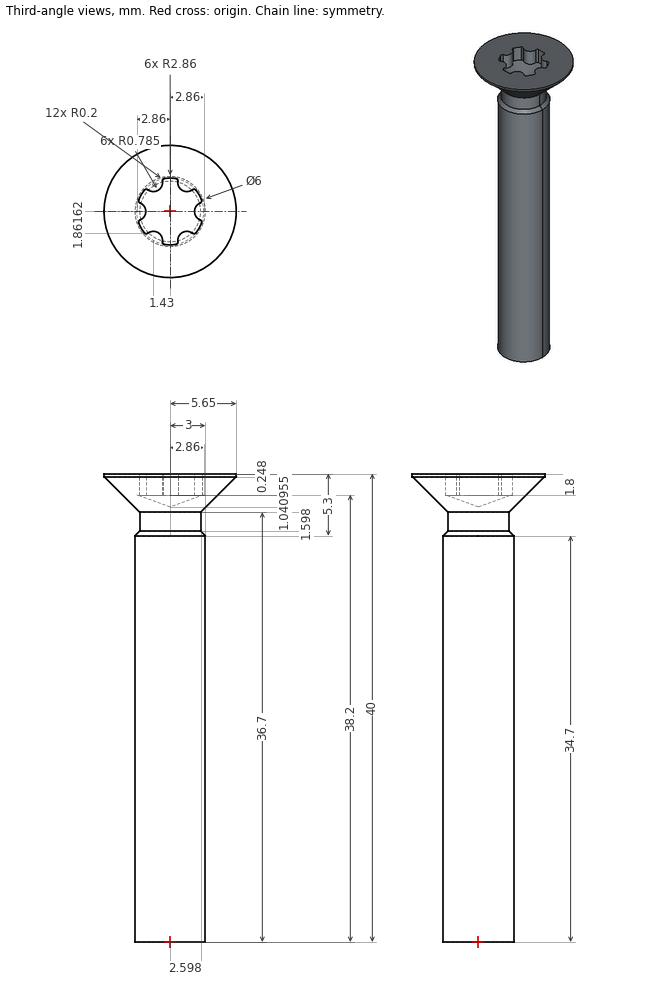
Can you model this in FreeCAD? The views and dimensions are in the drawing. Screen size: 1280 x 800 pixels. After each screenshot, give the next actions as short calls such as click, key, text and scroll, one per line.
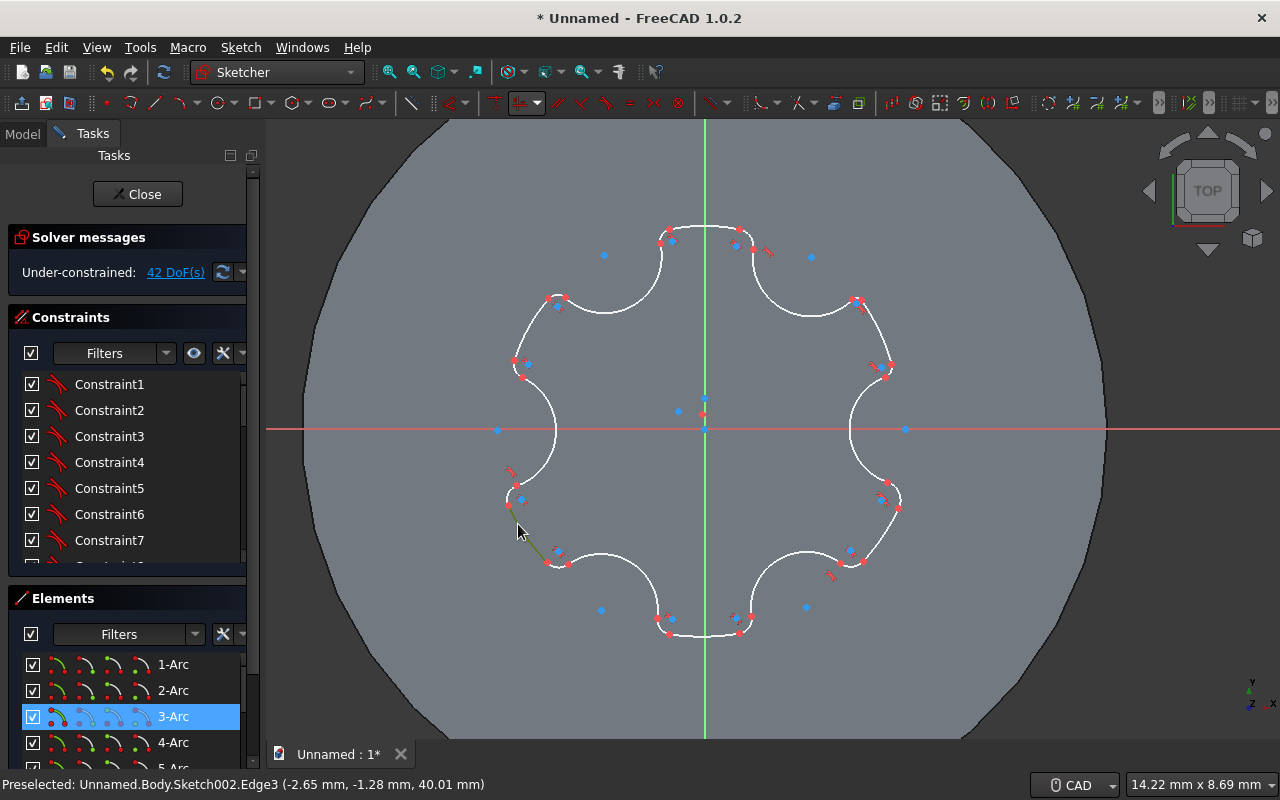
click(719, 226)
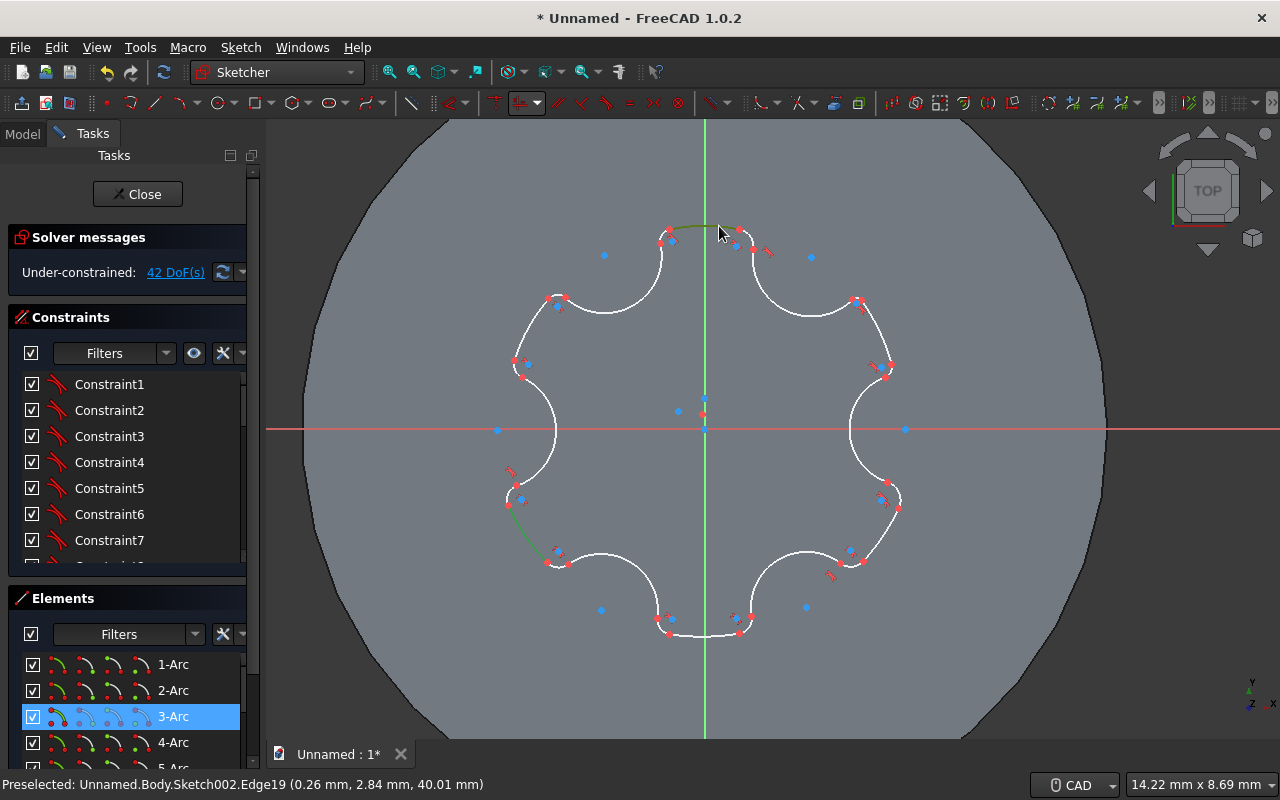
key(c)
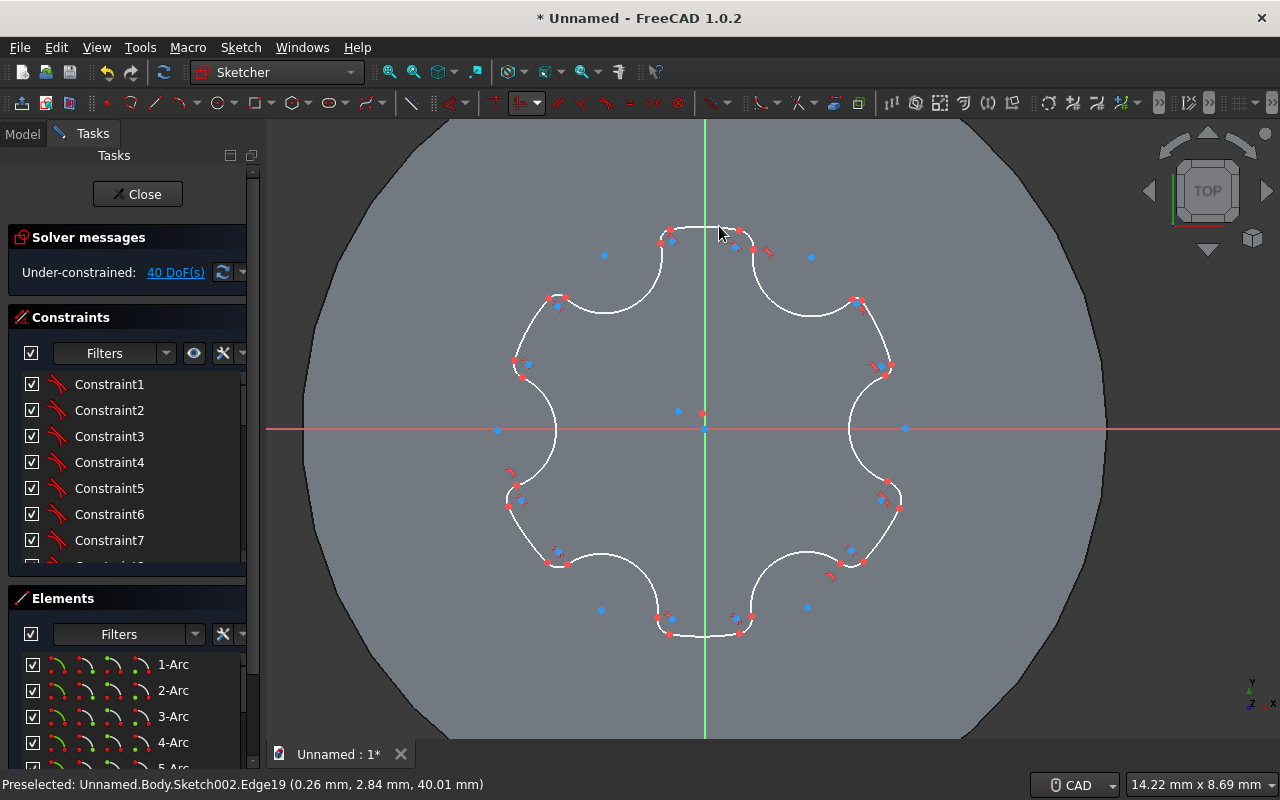
click(518, 525)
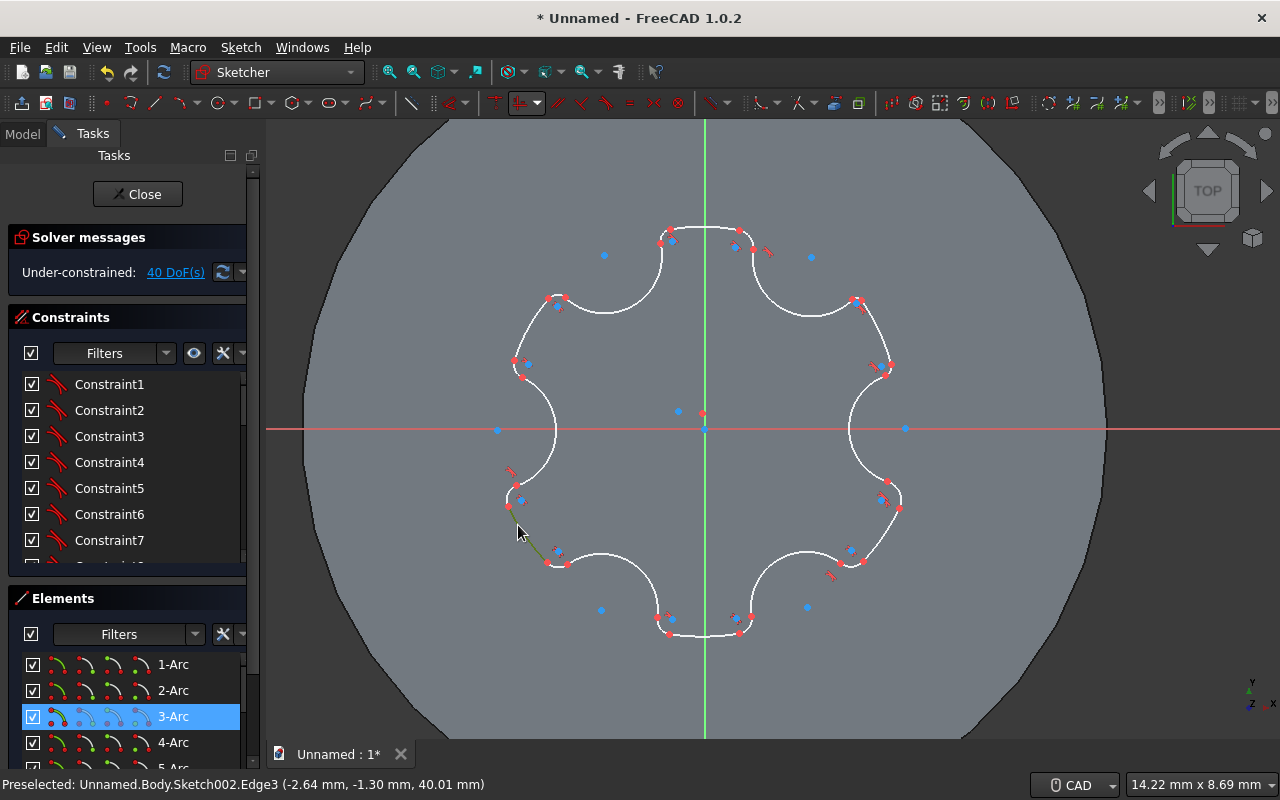
click(536, 316)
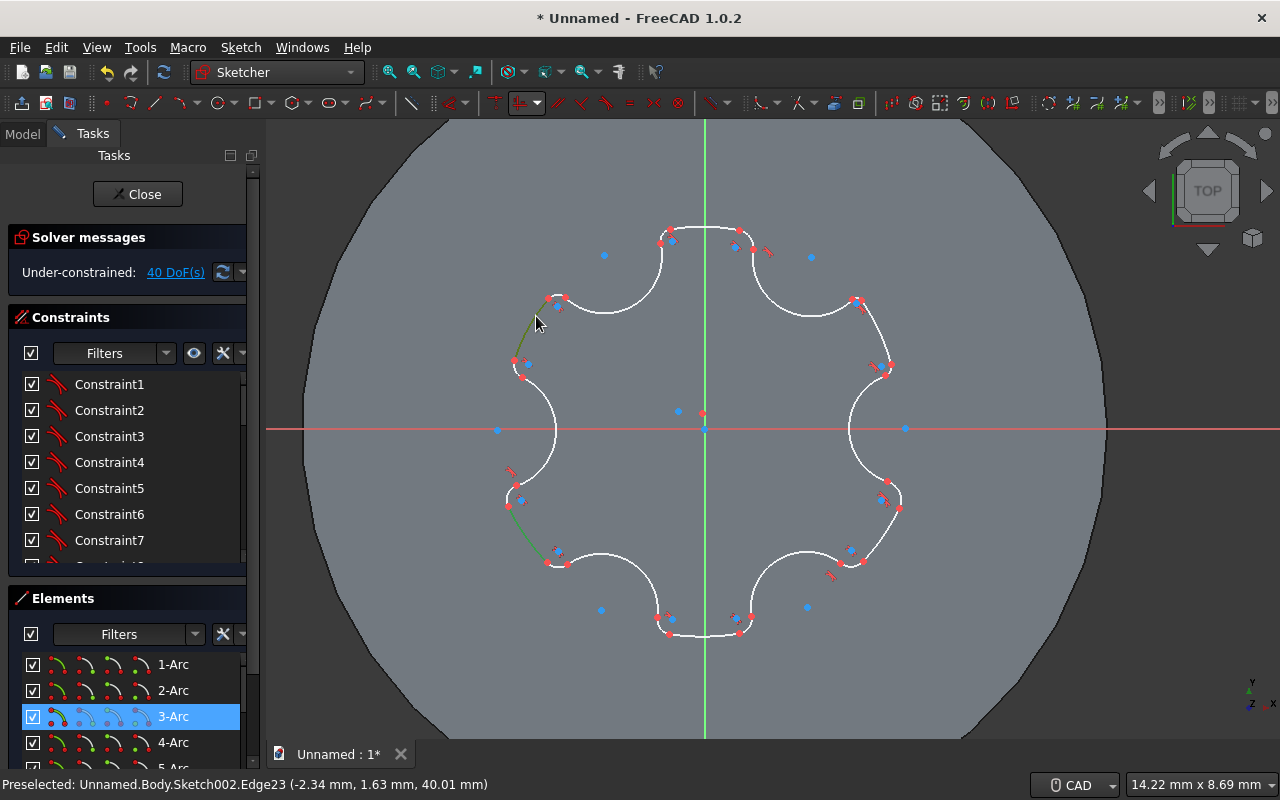
key(c)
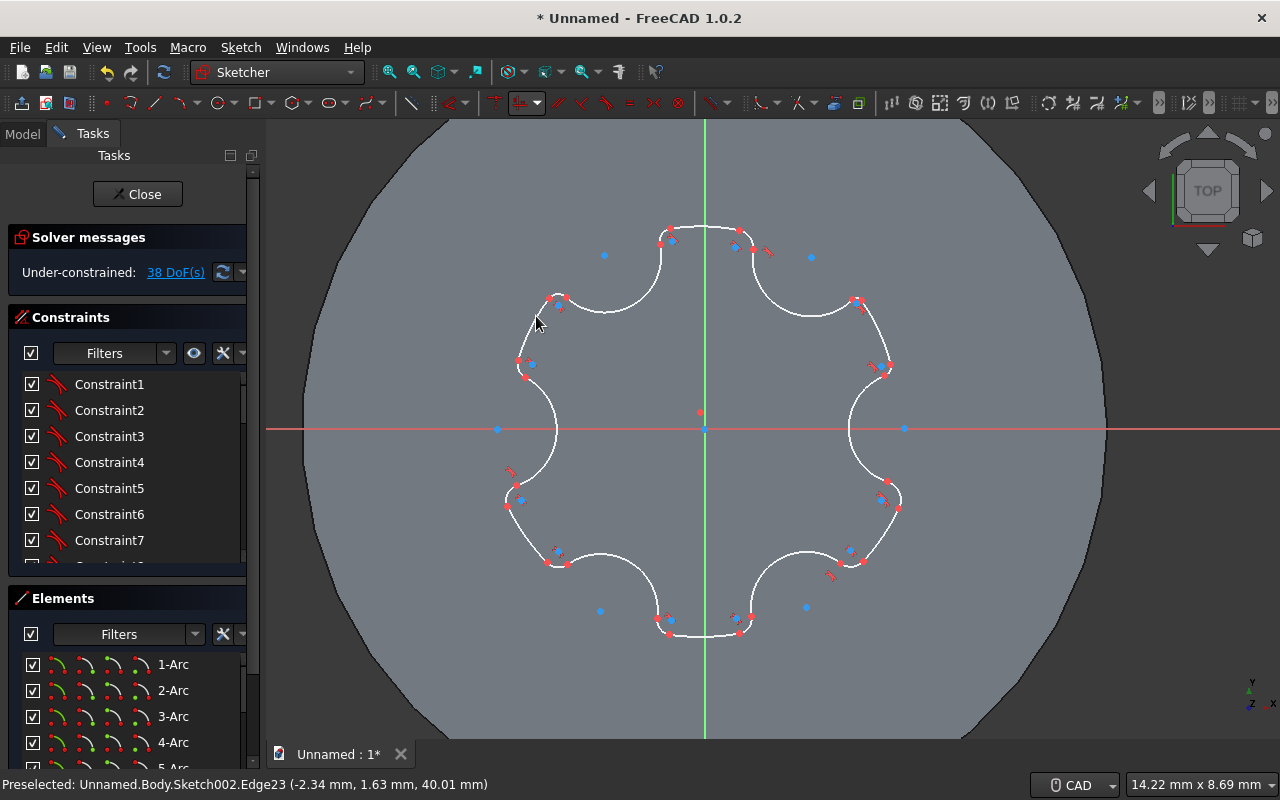
scroll(703, 421, up, 10)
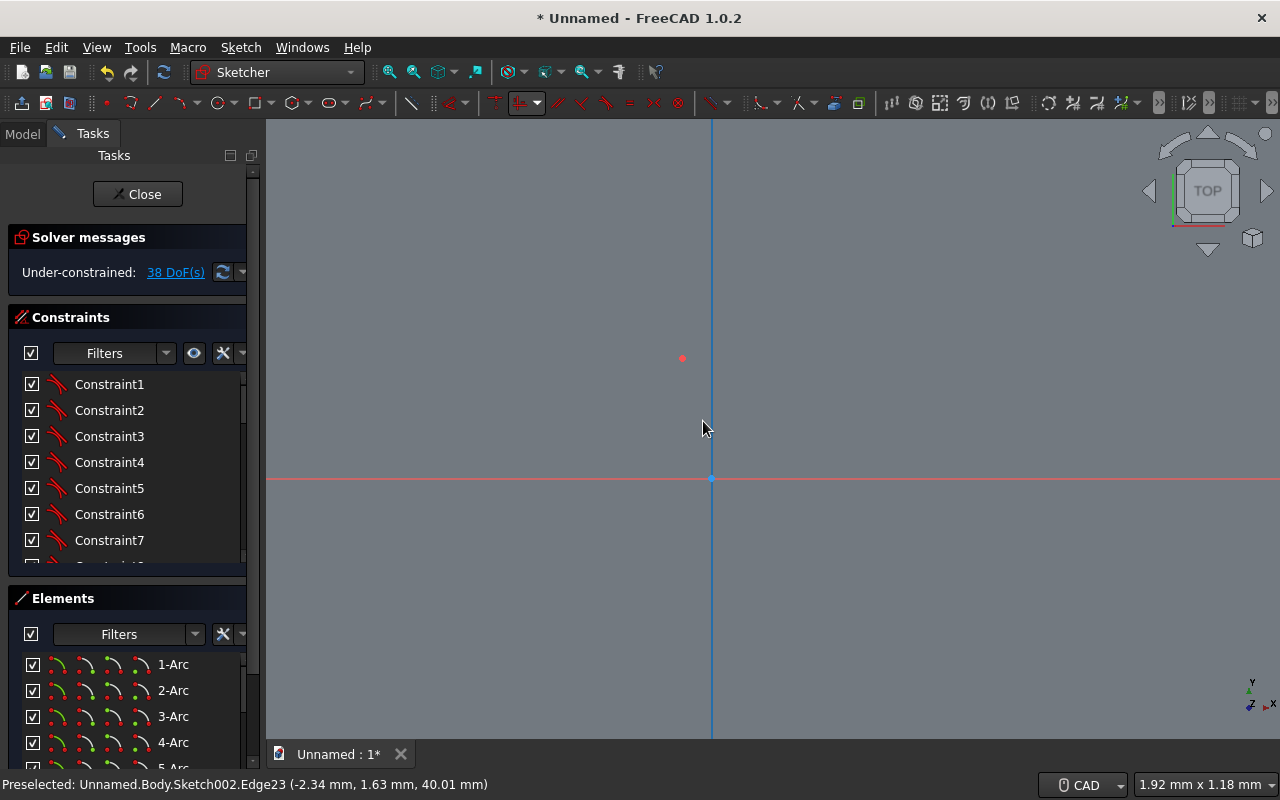
drag(672, 349, 722, 489)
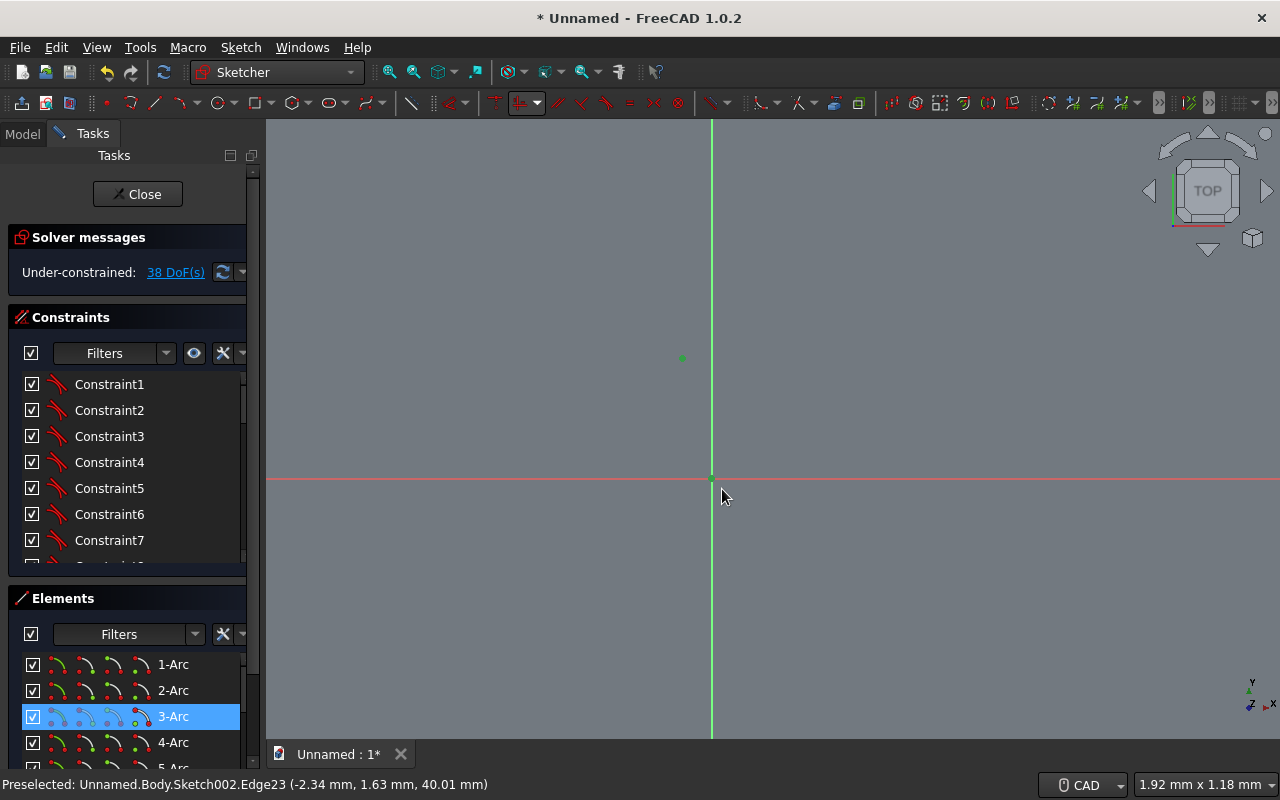
click(496, 104)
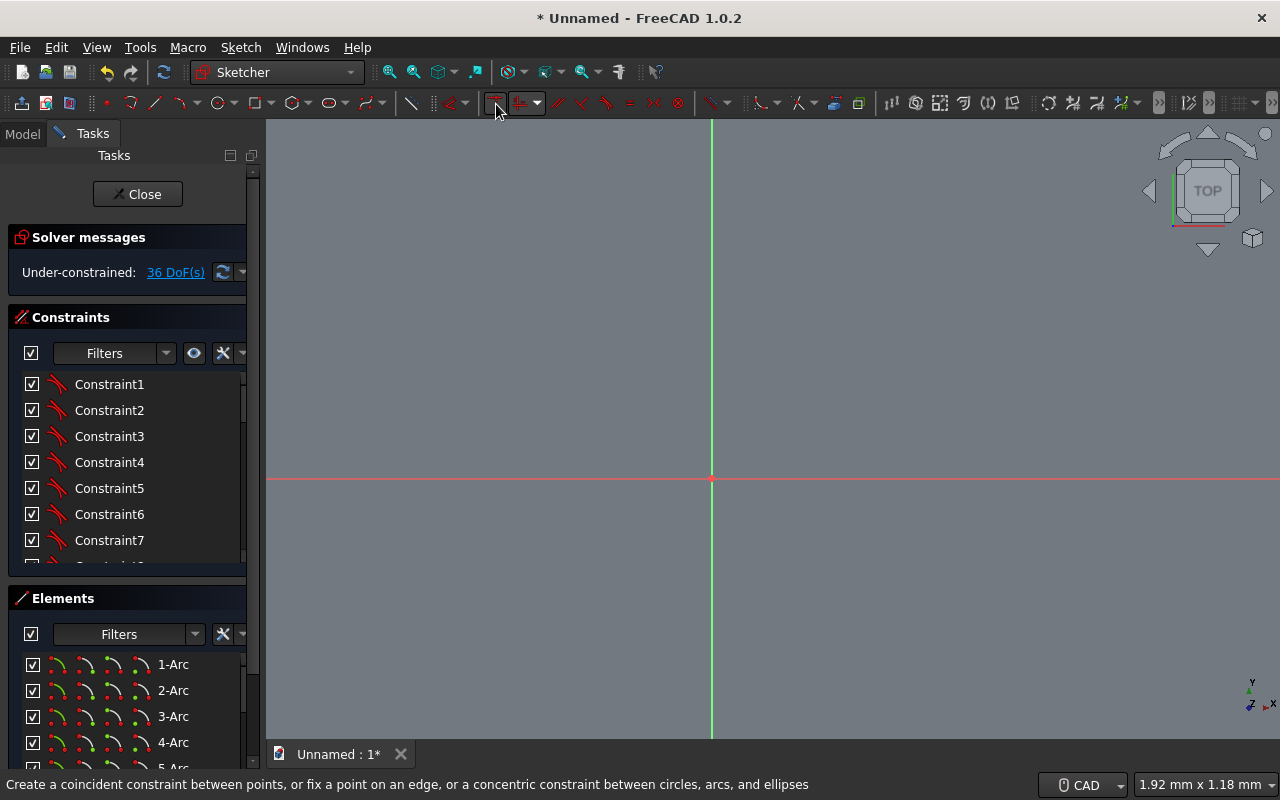
scroll(703, 421, down, 10)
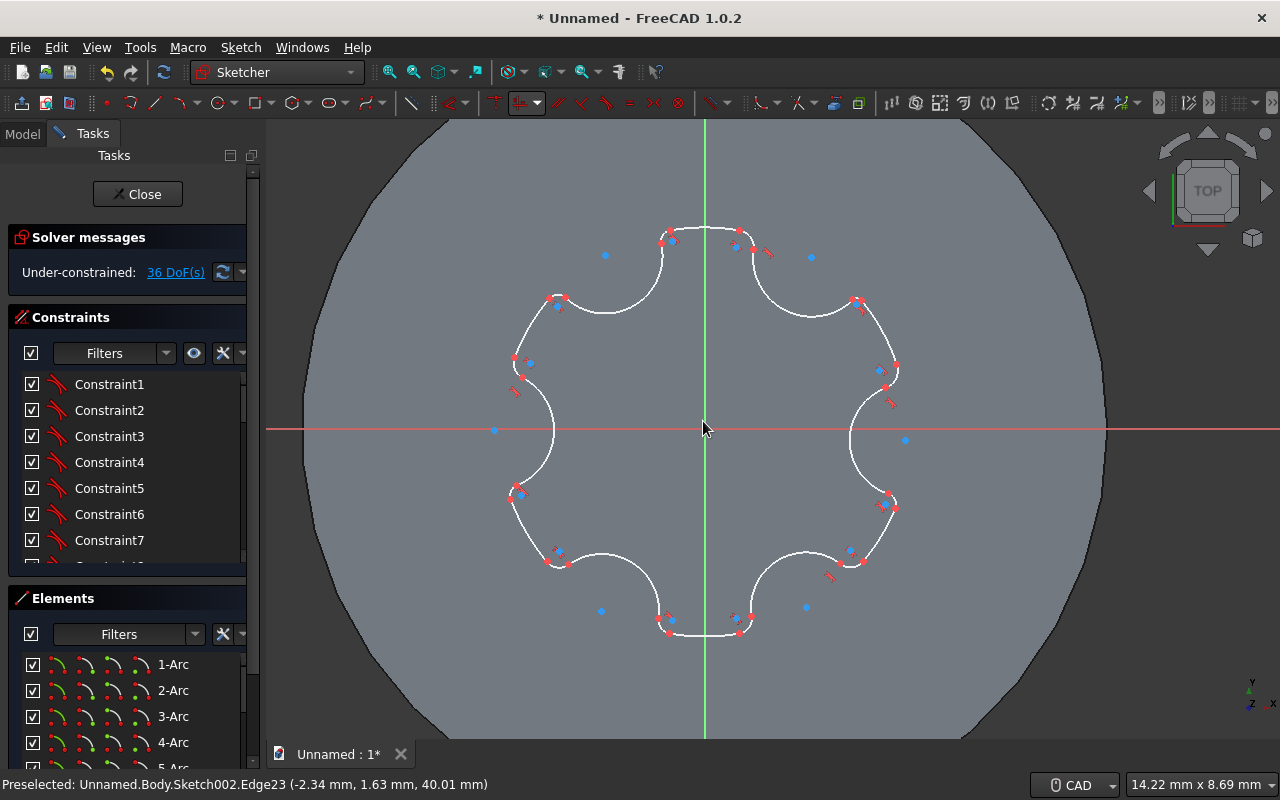
scroll(513, 488, up, 6)